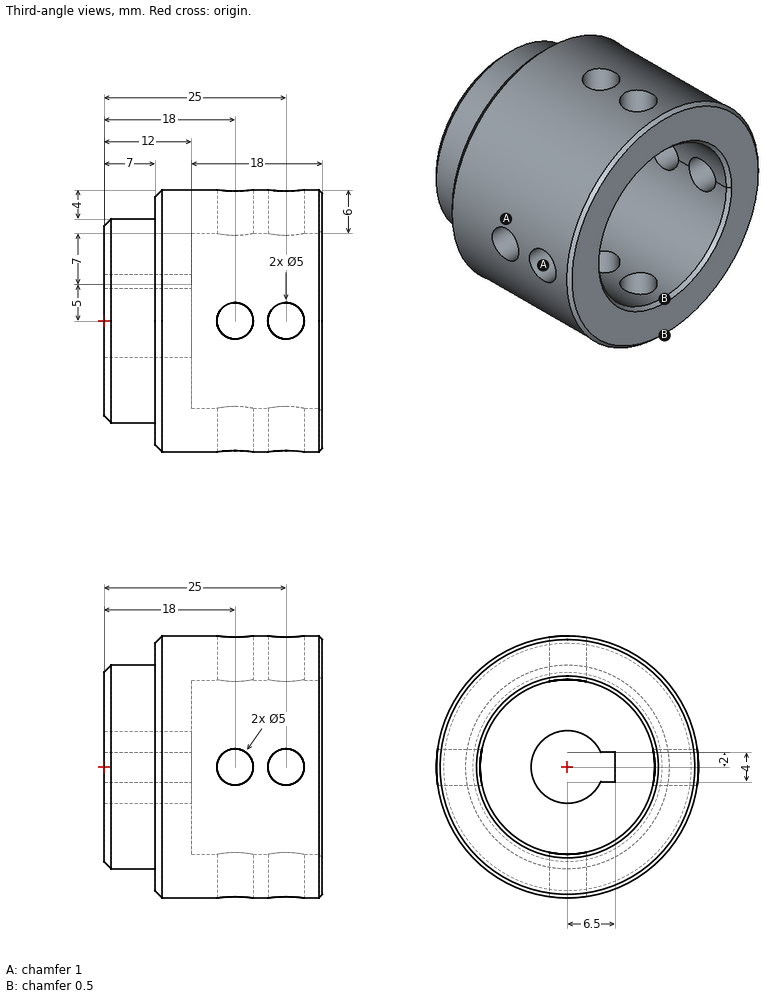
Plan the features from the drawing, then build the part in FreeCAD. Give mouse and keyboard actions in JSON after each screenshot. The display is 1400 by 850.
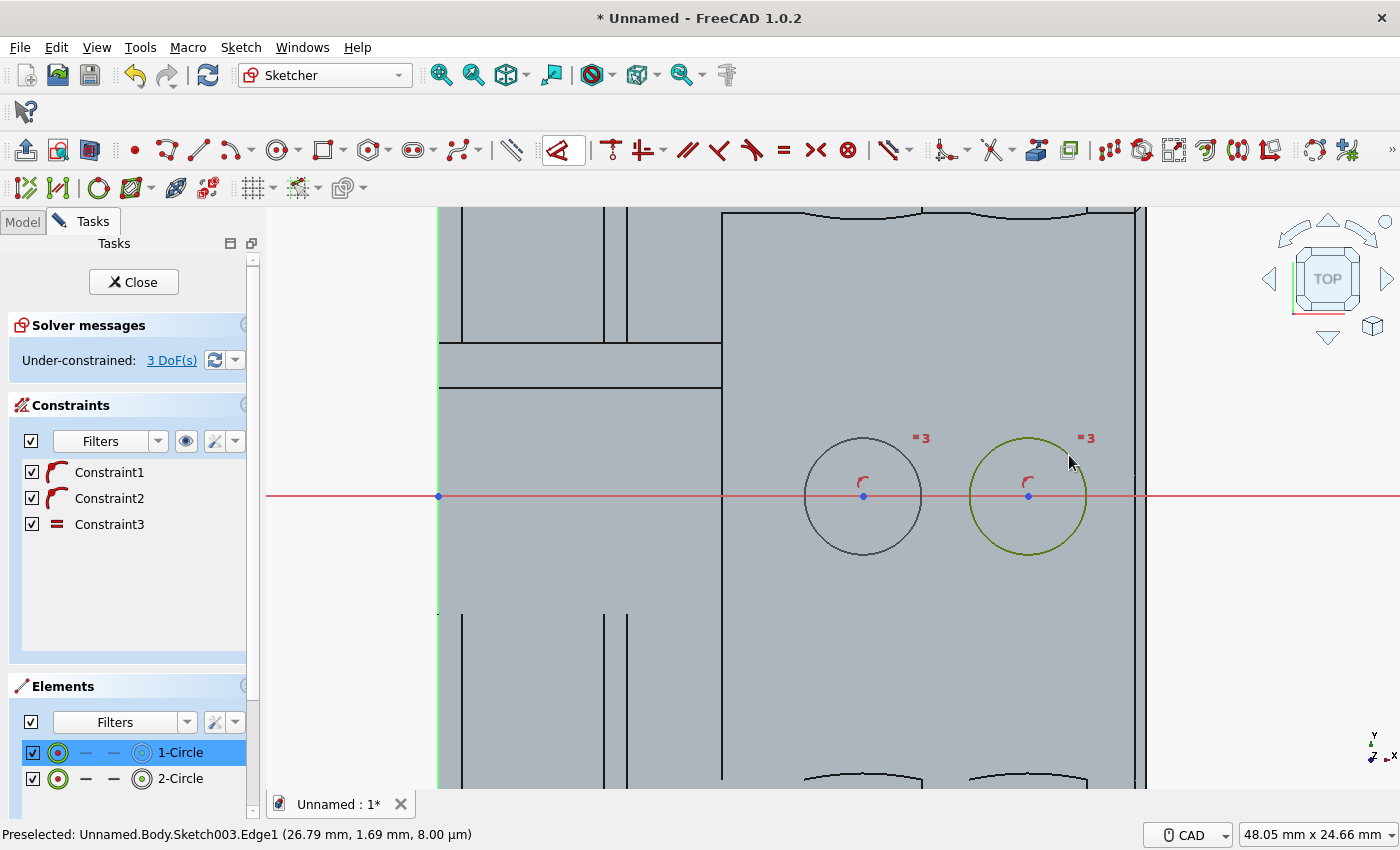
{"action": "key", "text": "k o"}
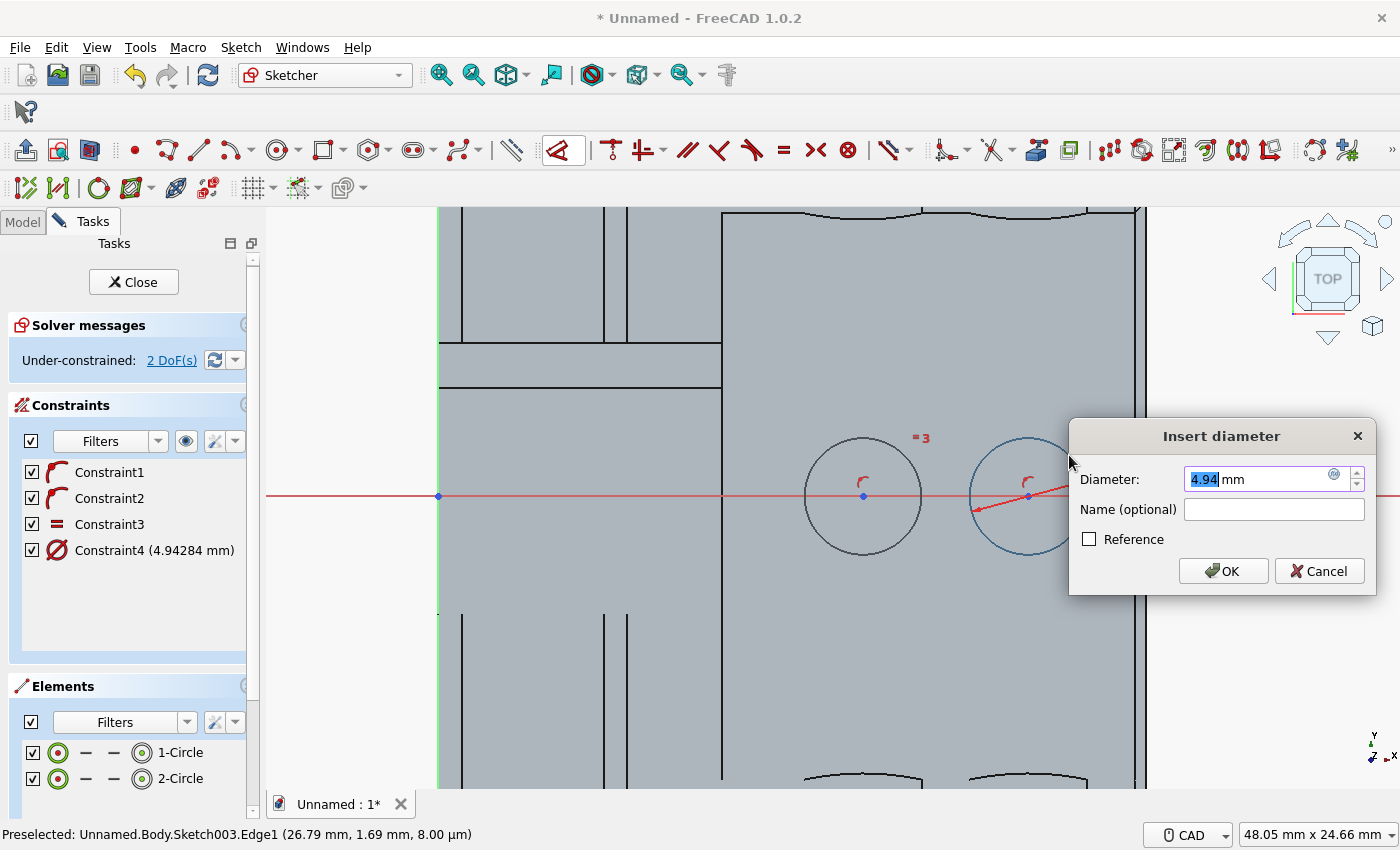
{"action": "type", "text": "5"}
{"action": "key", "text": "Return"}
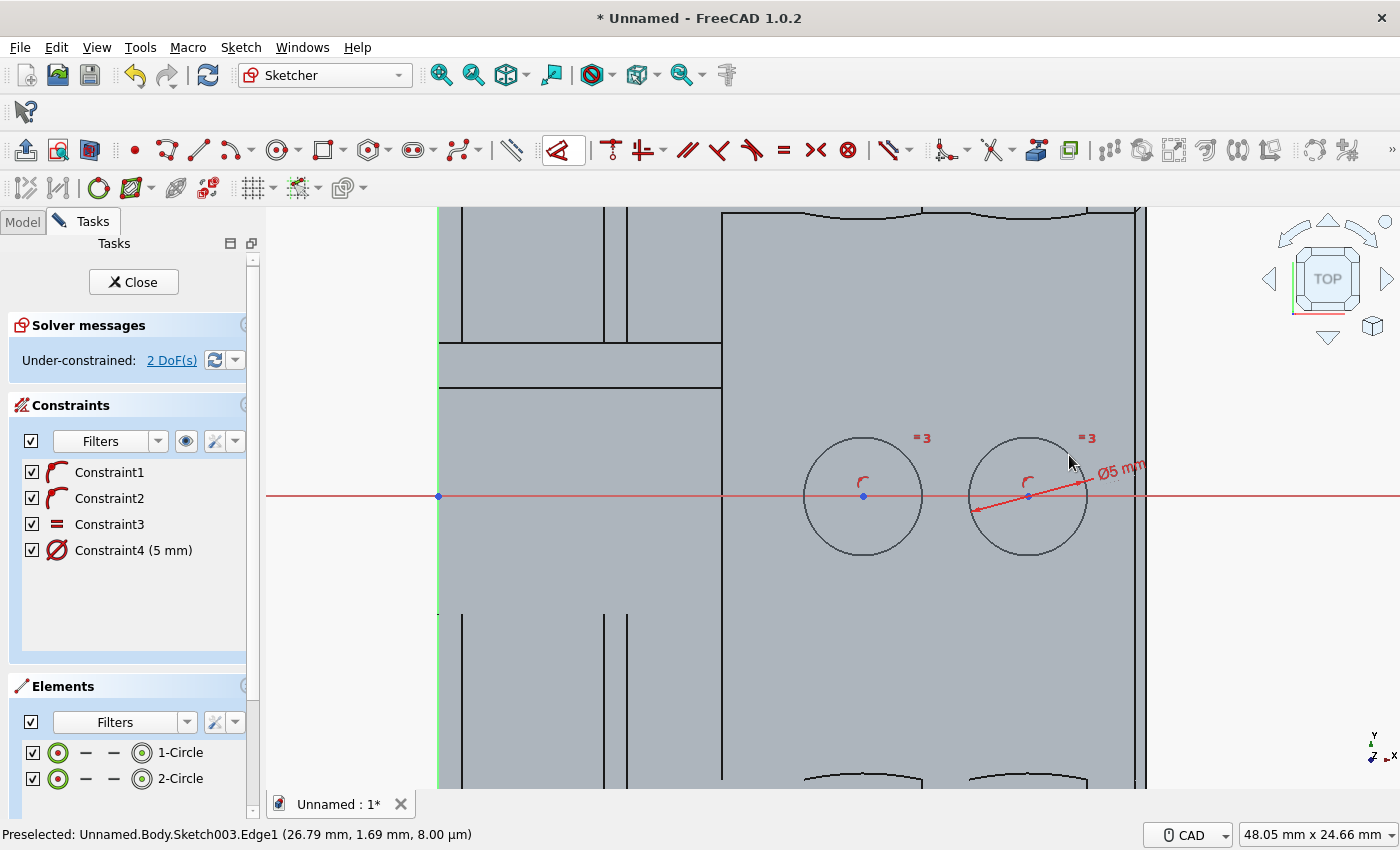
{"action": "left_click", "coordinate": [1028, 496]}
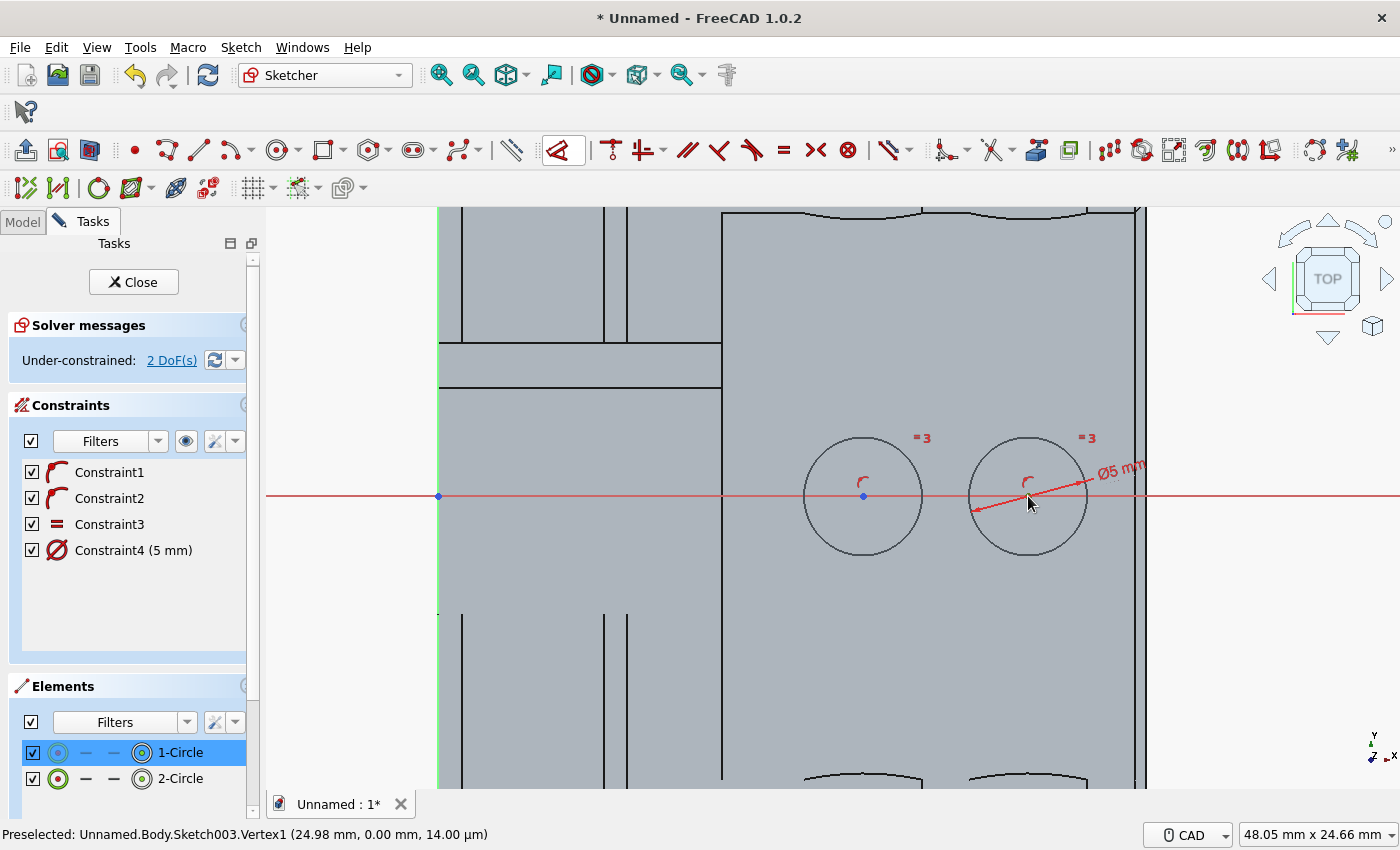
{"action": "left_click", "coordinate": [580, 150]}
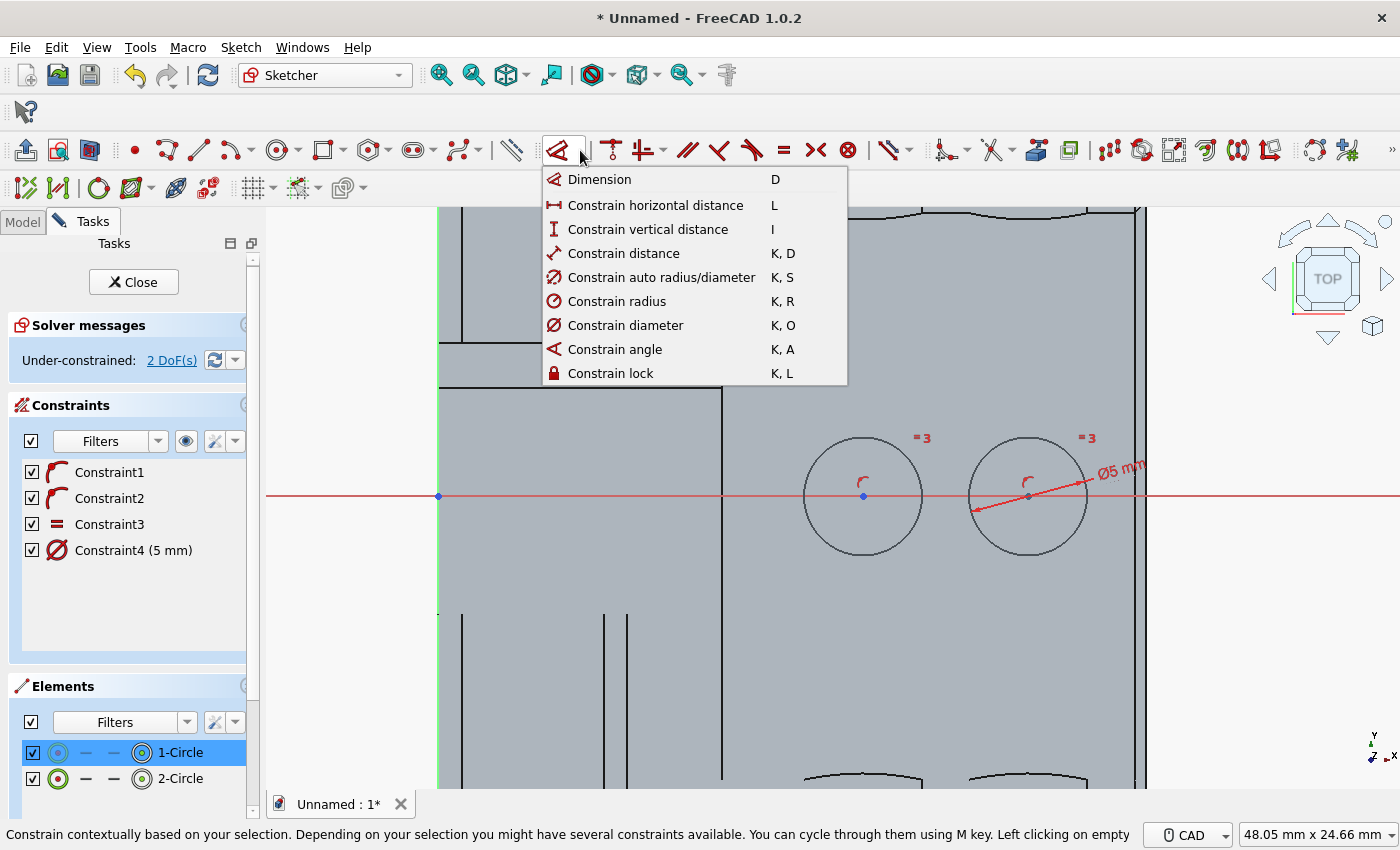
{"action": "left_click", "coordinate": [695, 205]}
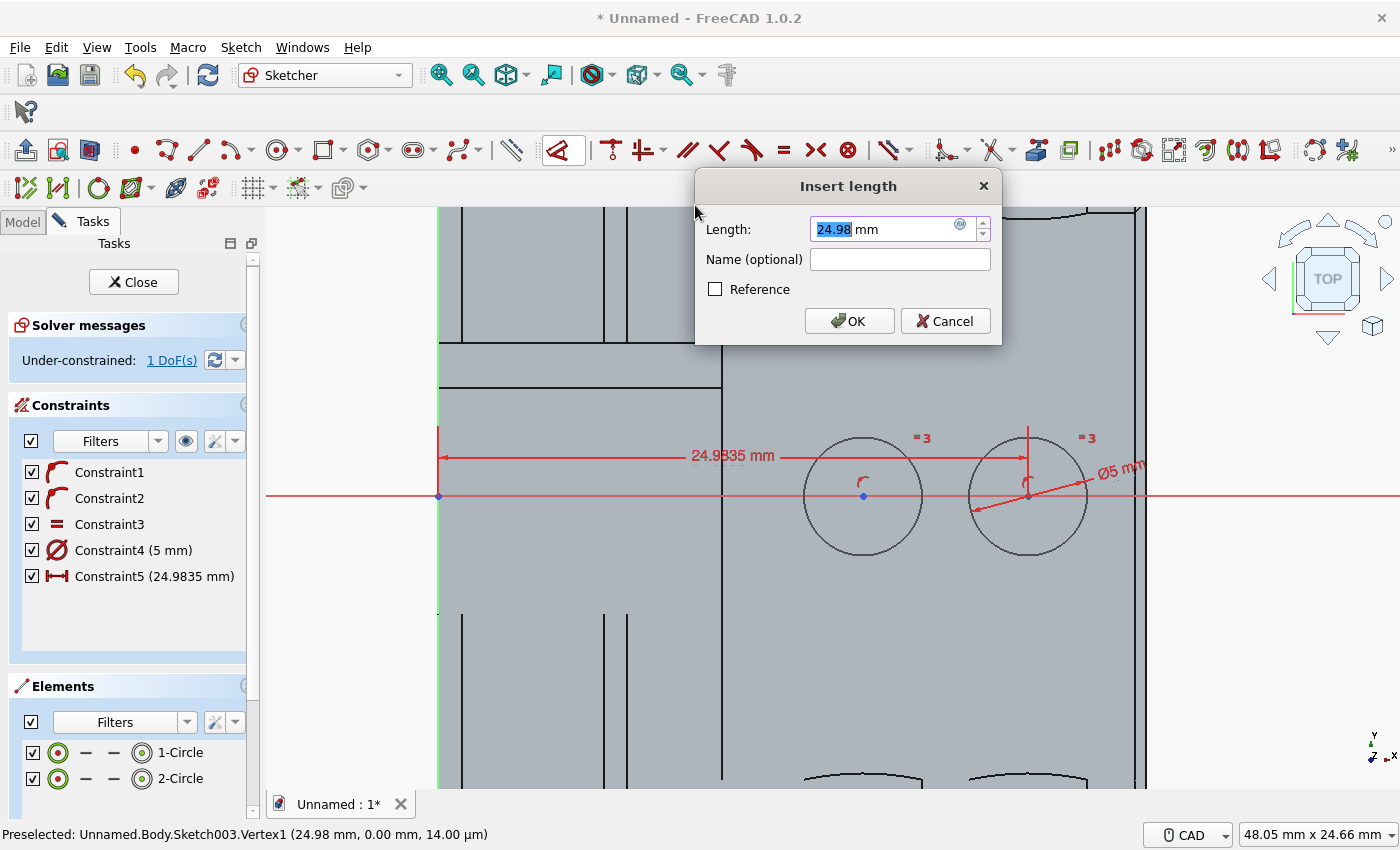
{"action": "type", "text": "25"}
{"action": "key", "text": "Return"}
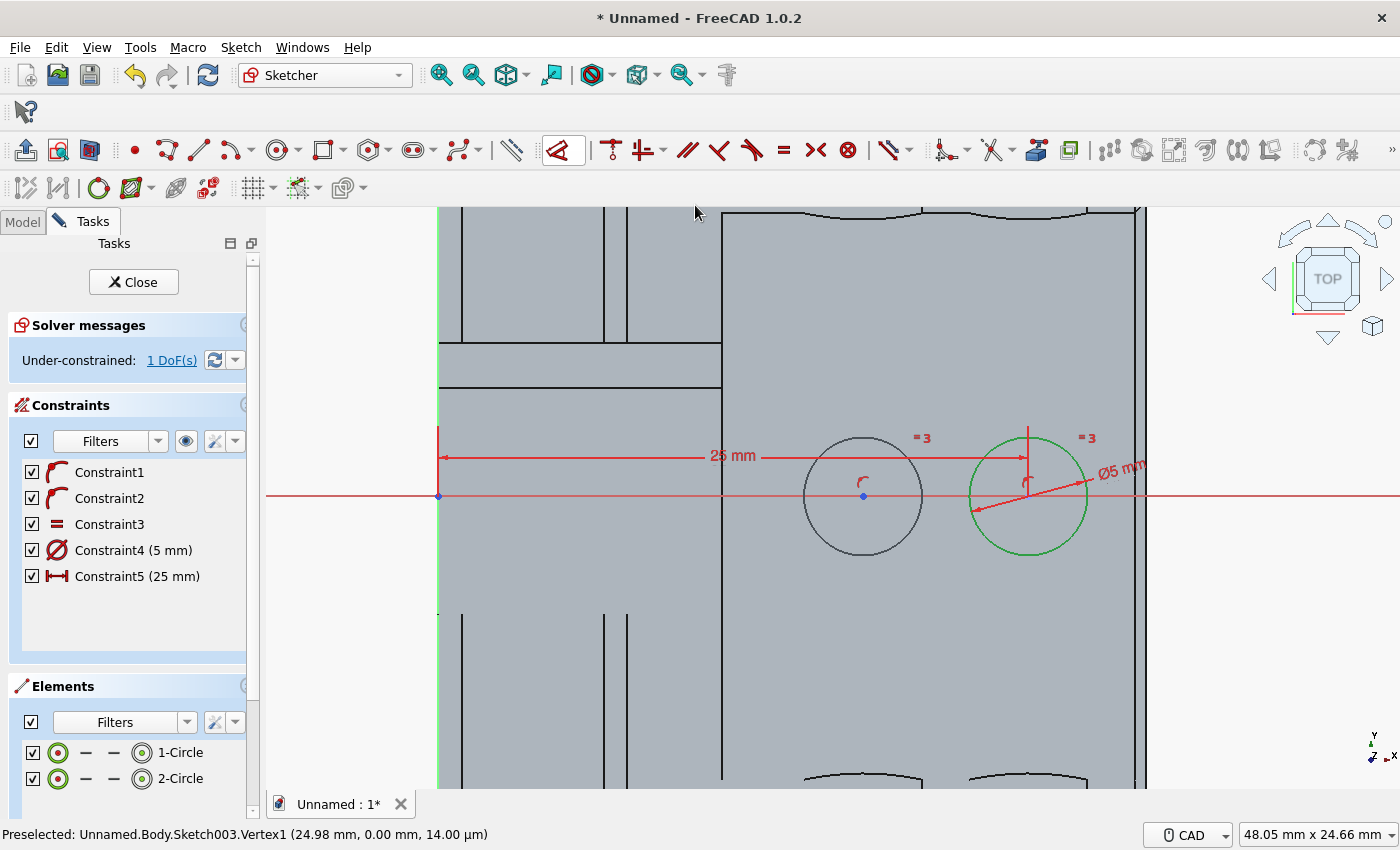
{"action": "left_click", "coordinate": [863, 496]}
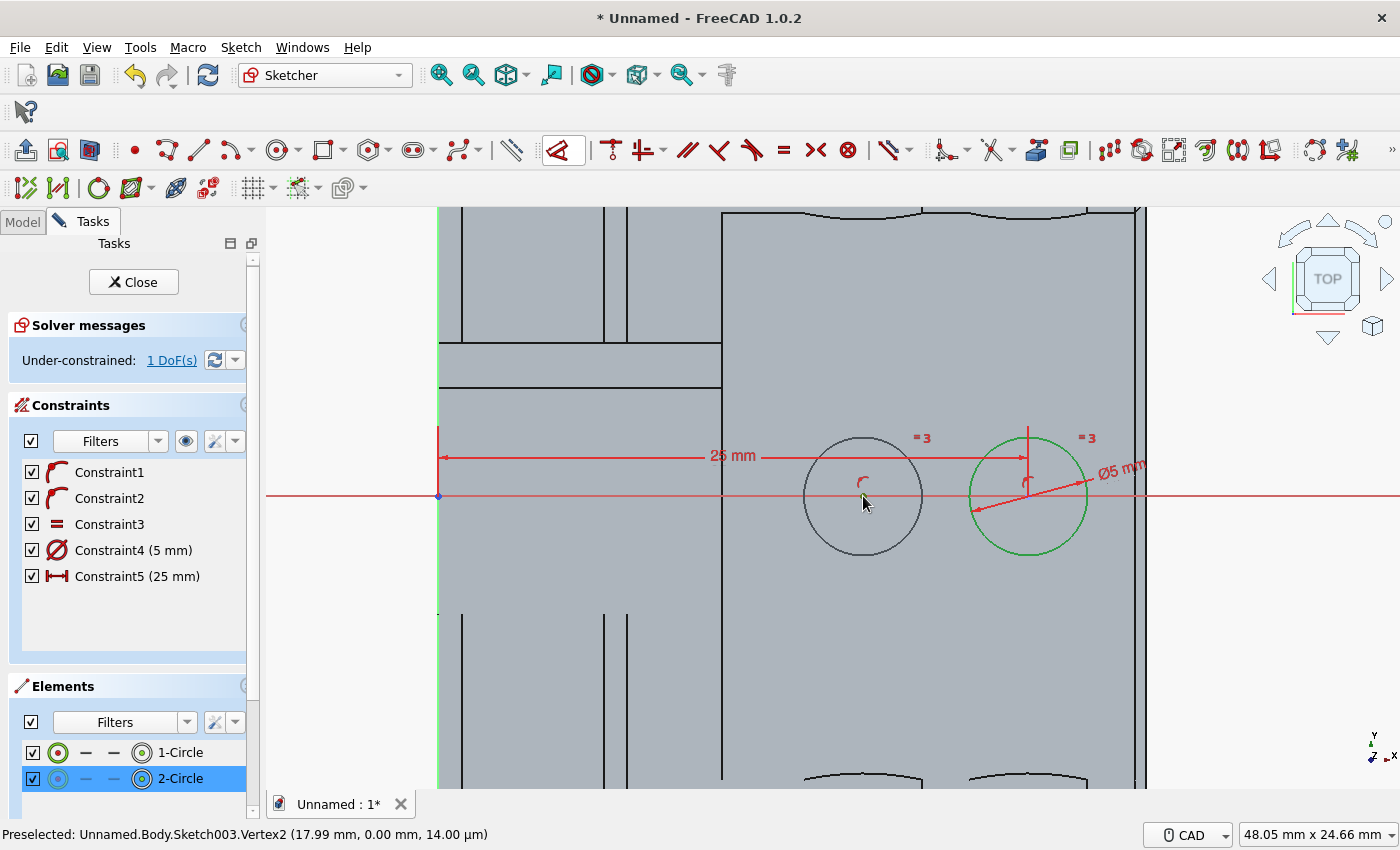
{"action": "key", "text": "l"}